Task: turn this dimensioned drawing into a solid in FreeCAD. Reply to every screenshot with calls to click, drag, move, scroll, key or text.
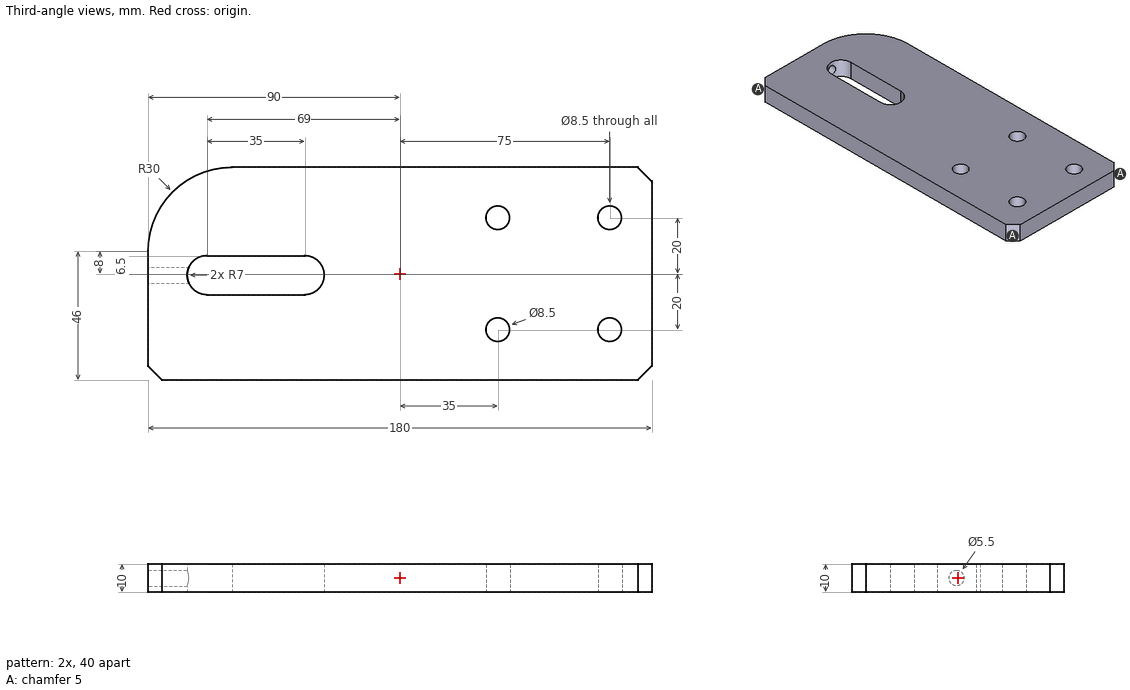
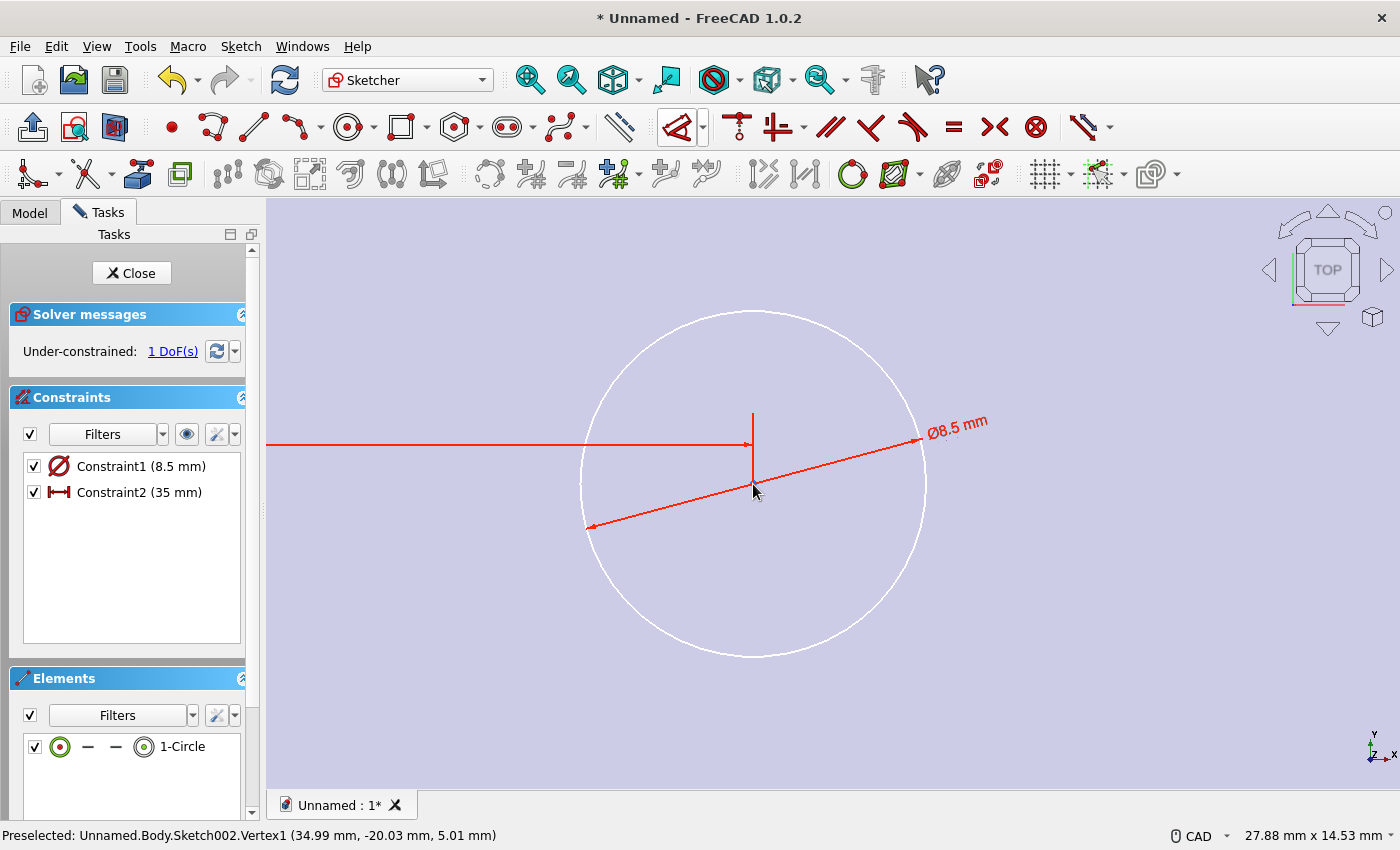
click(753, 484)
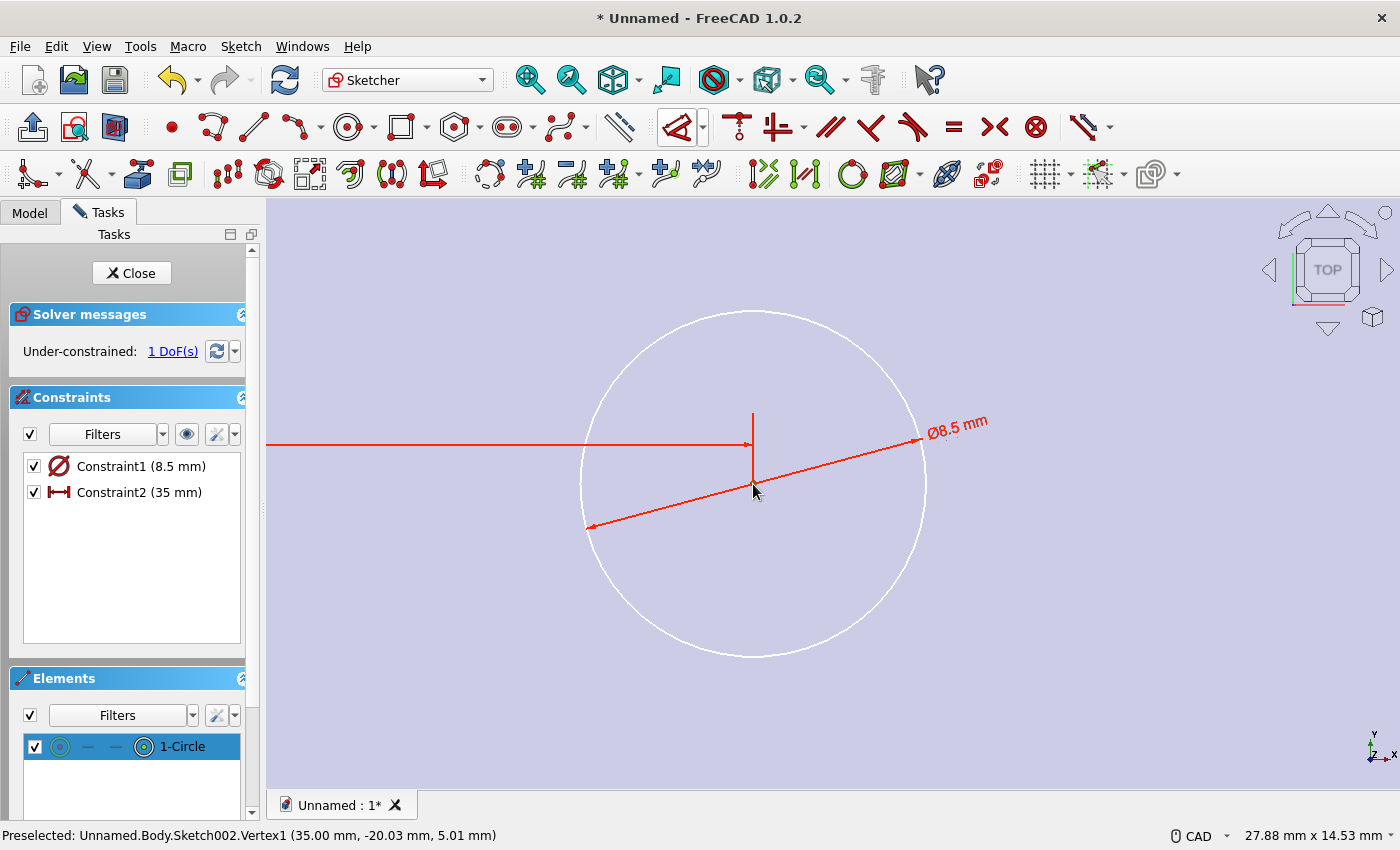
key(i)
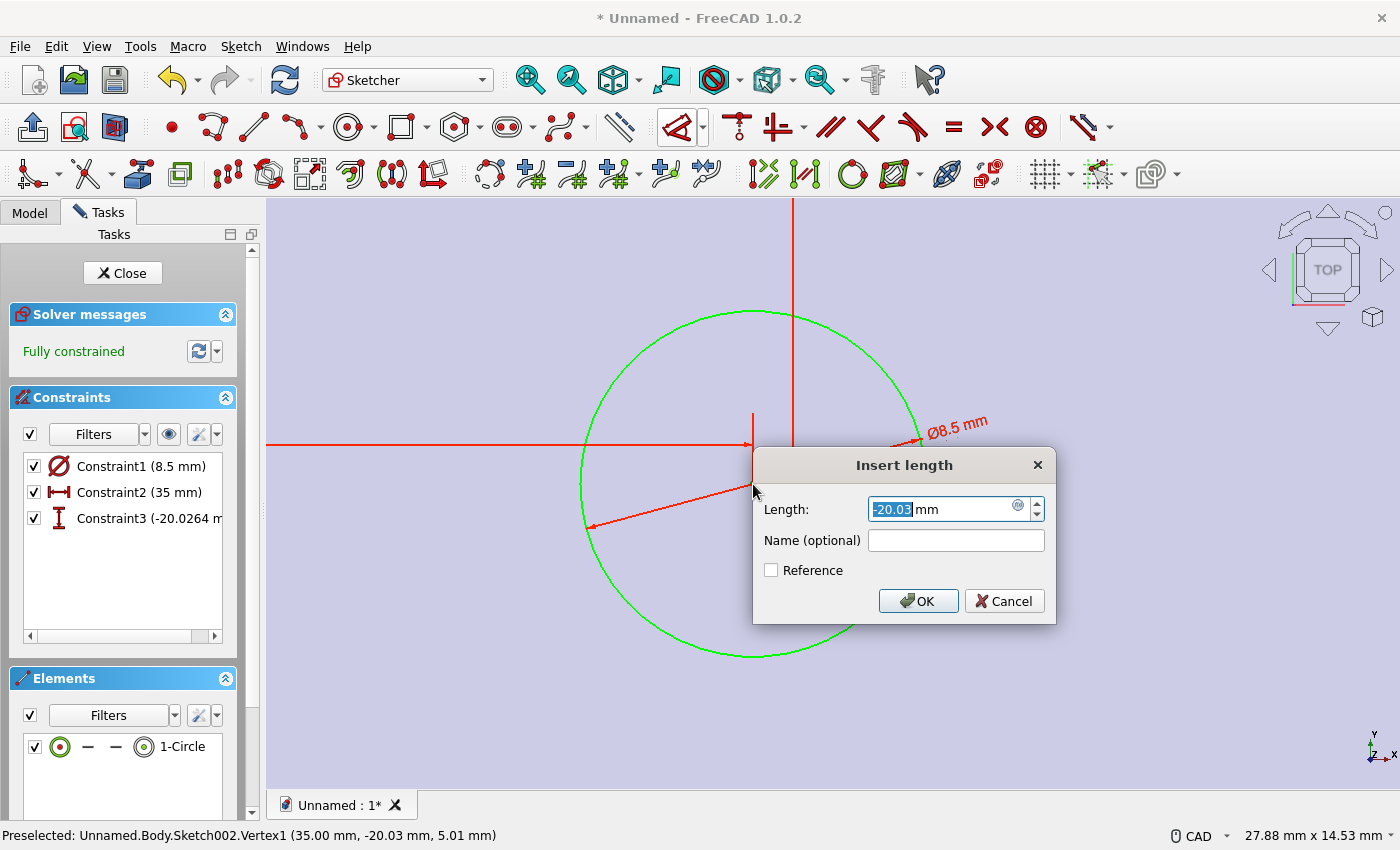
text(-20)
key(Return)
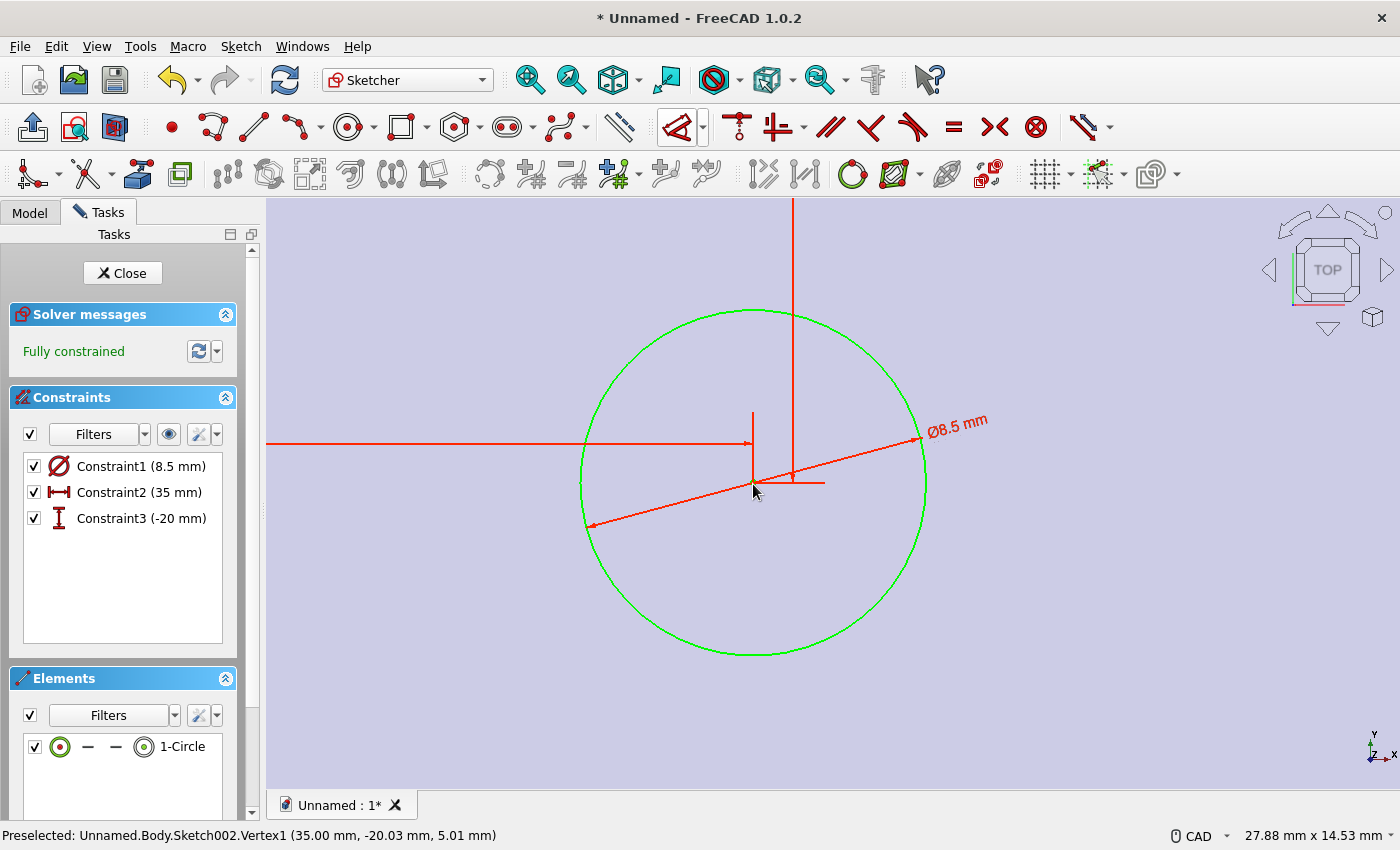
click(123, 273)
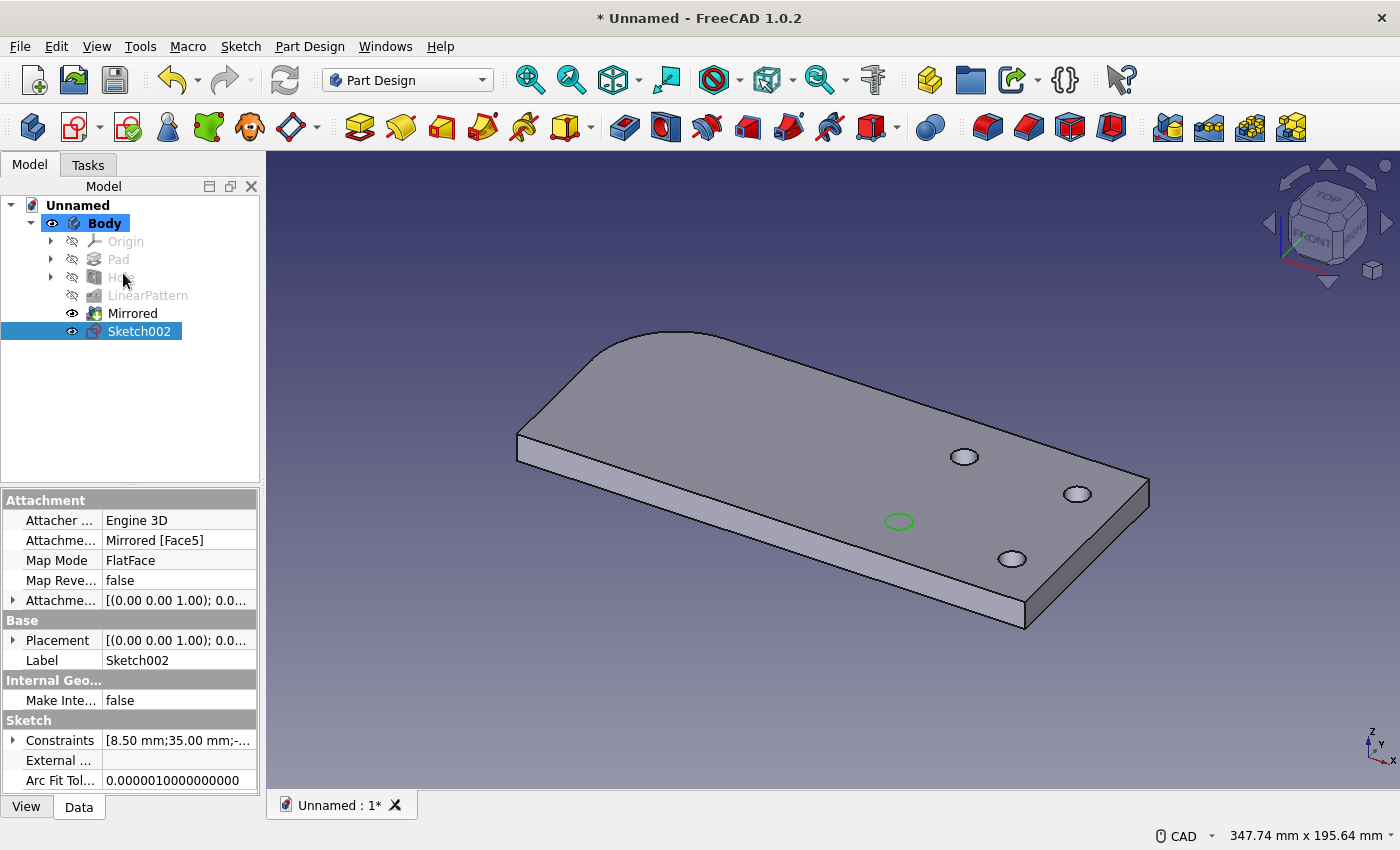
click(625, 128)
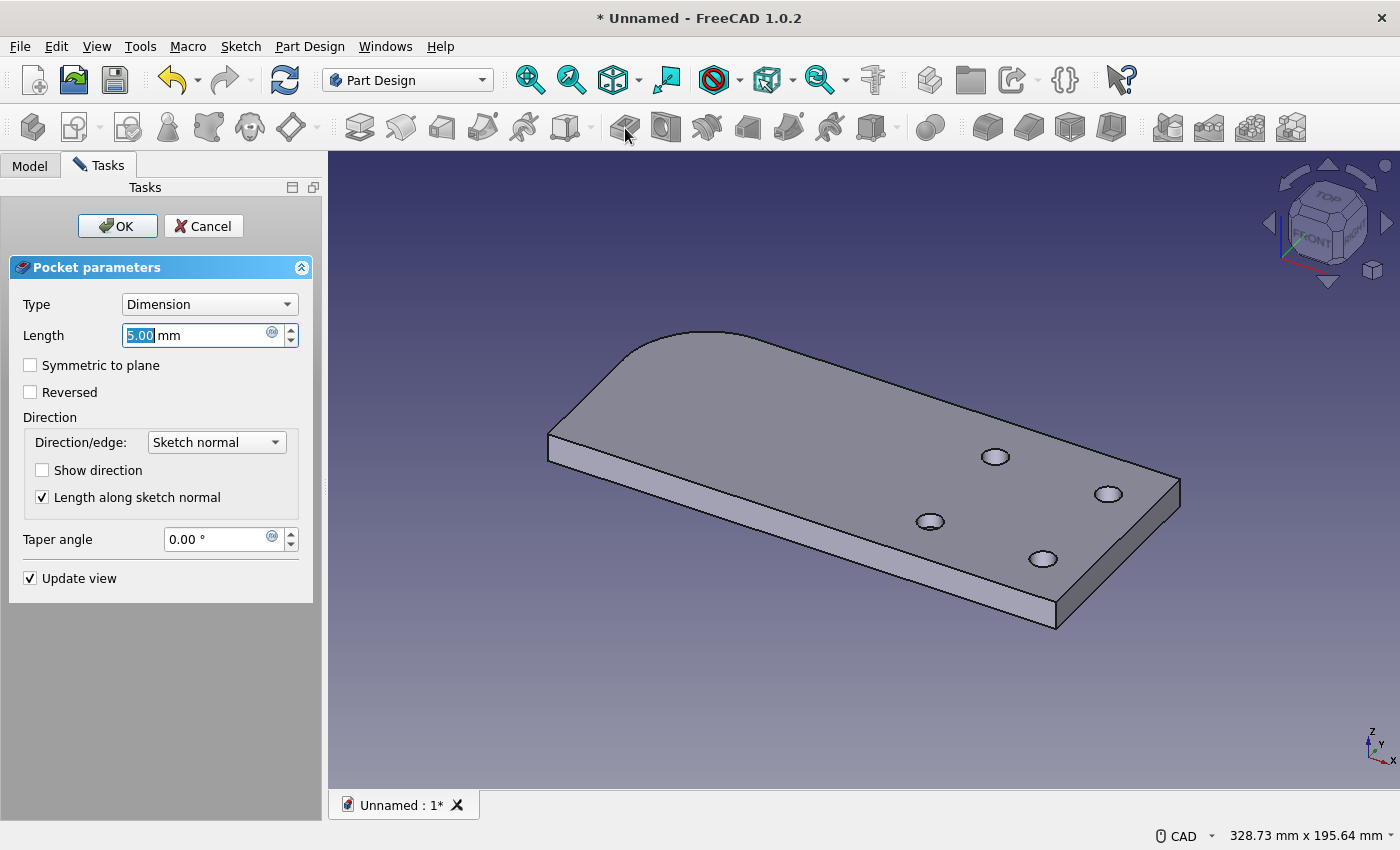
click(210, 304)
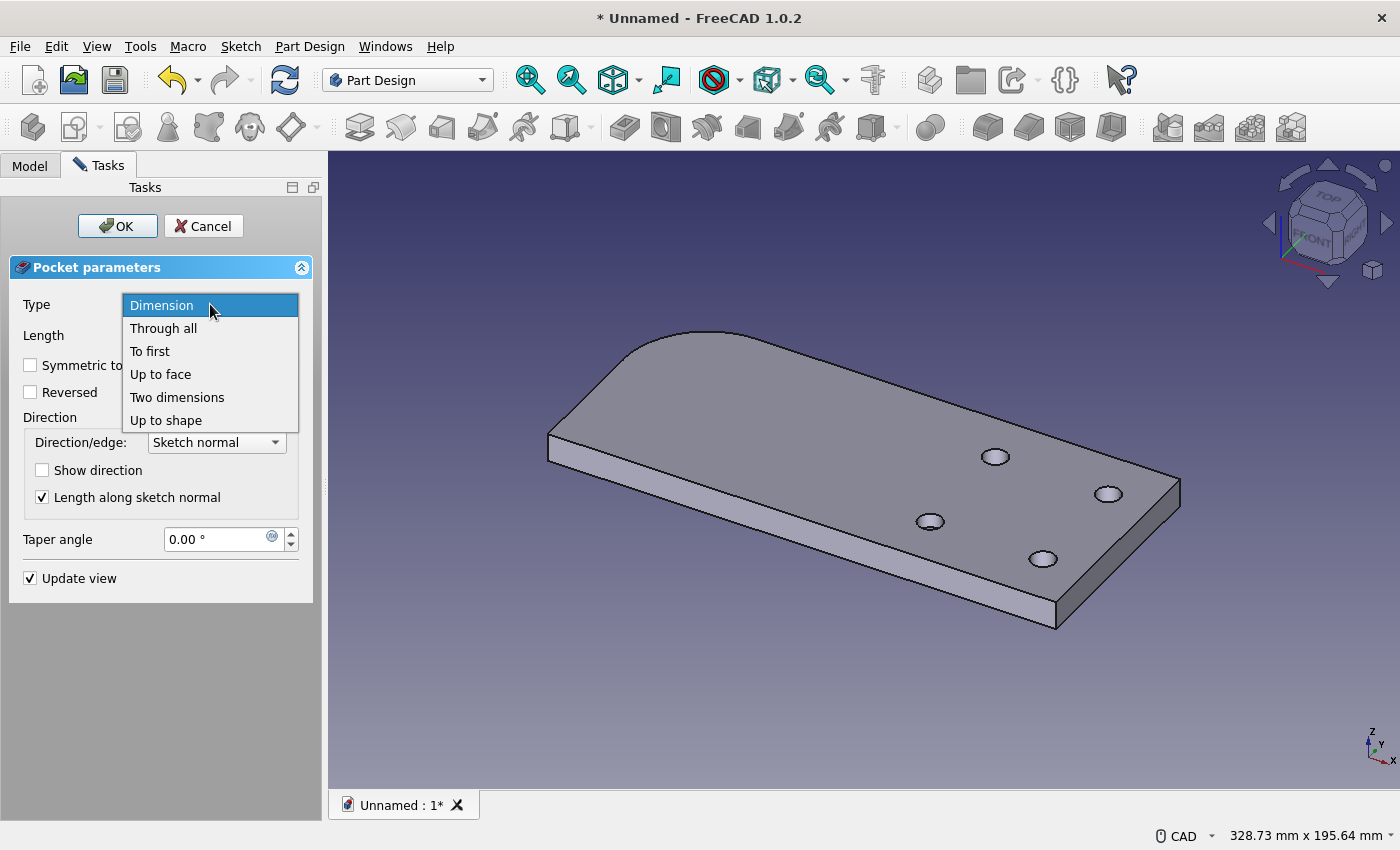
click(208, 328)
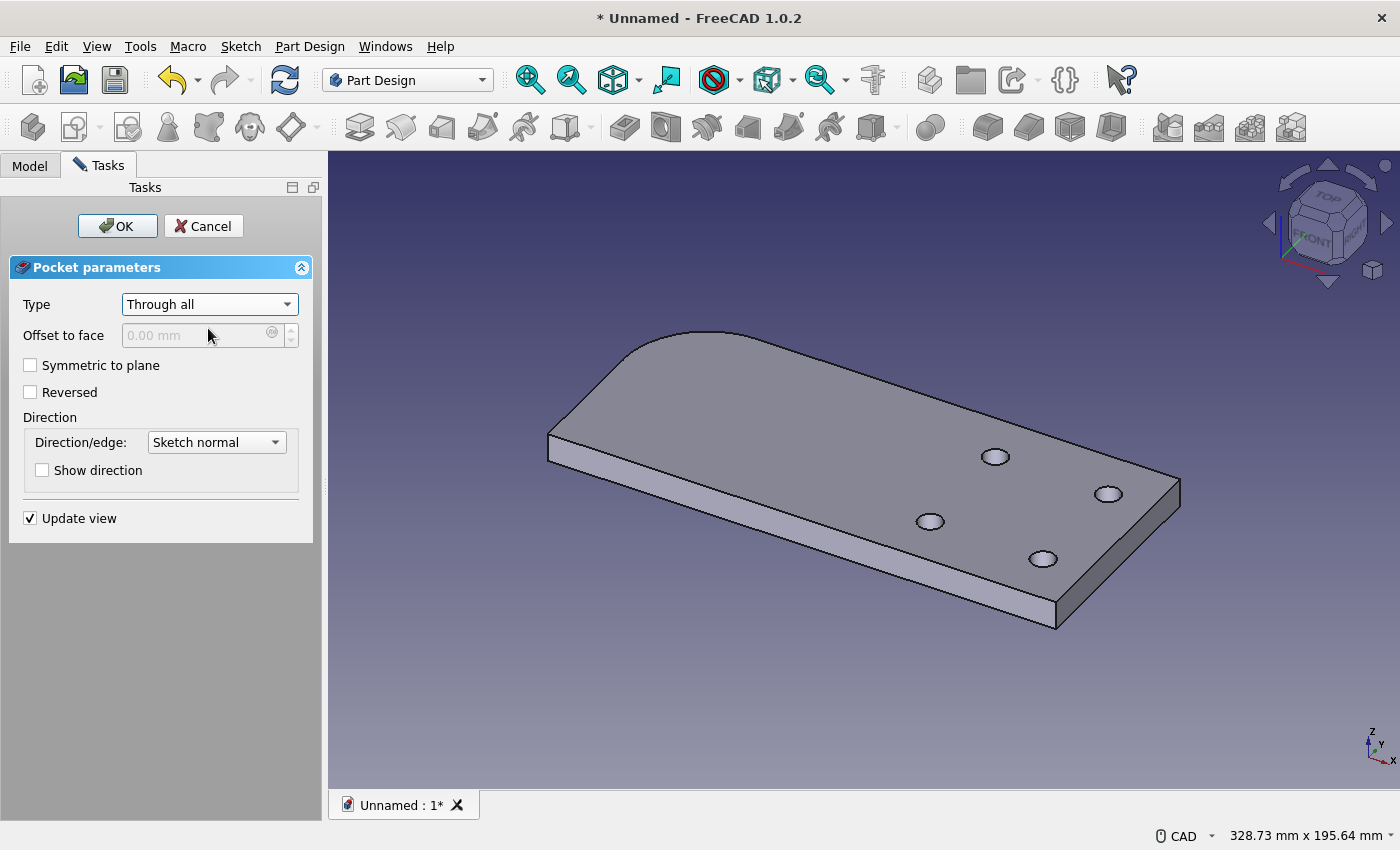
click(118, 226)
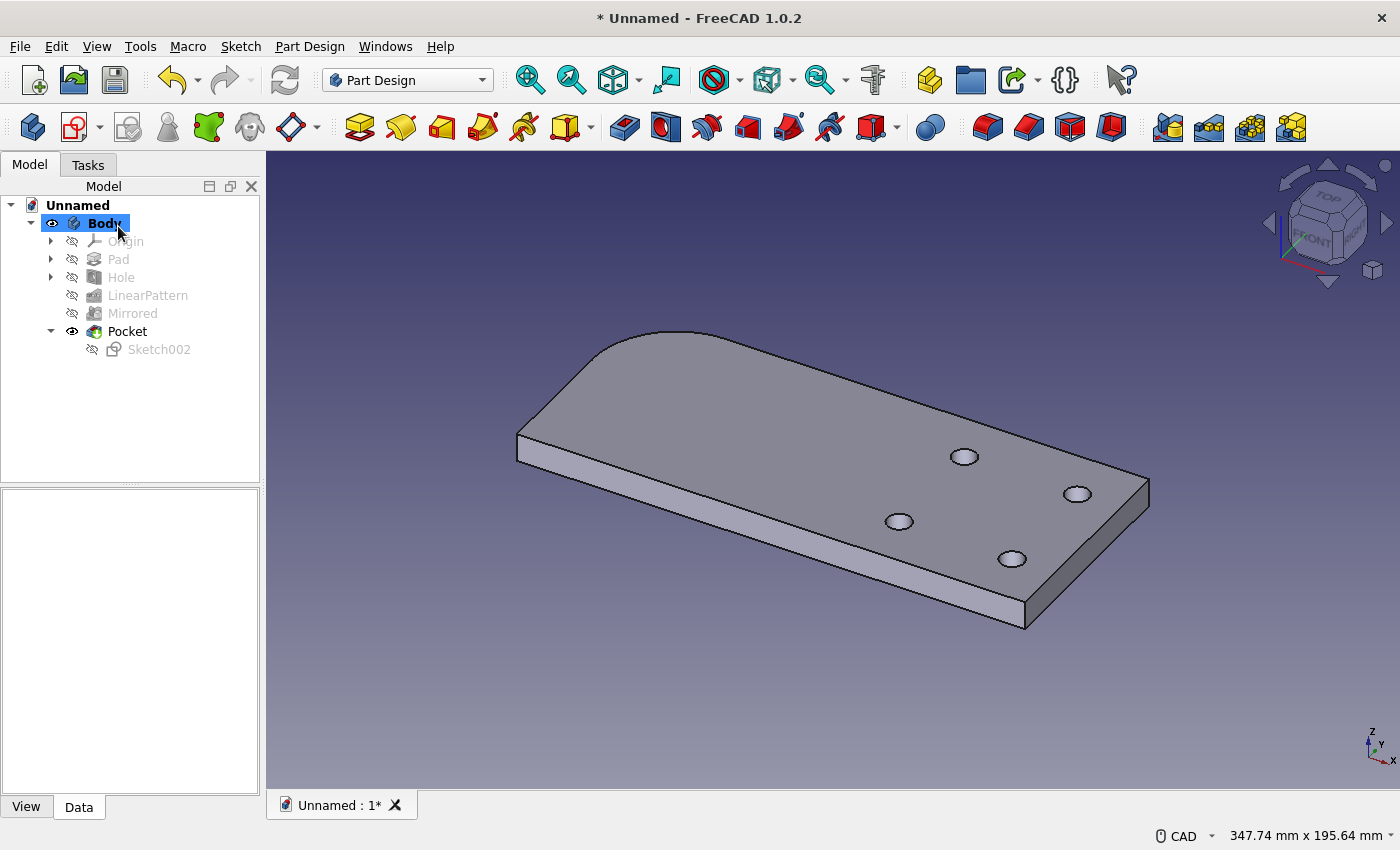
click(760, 432)